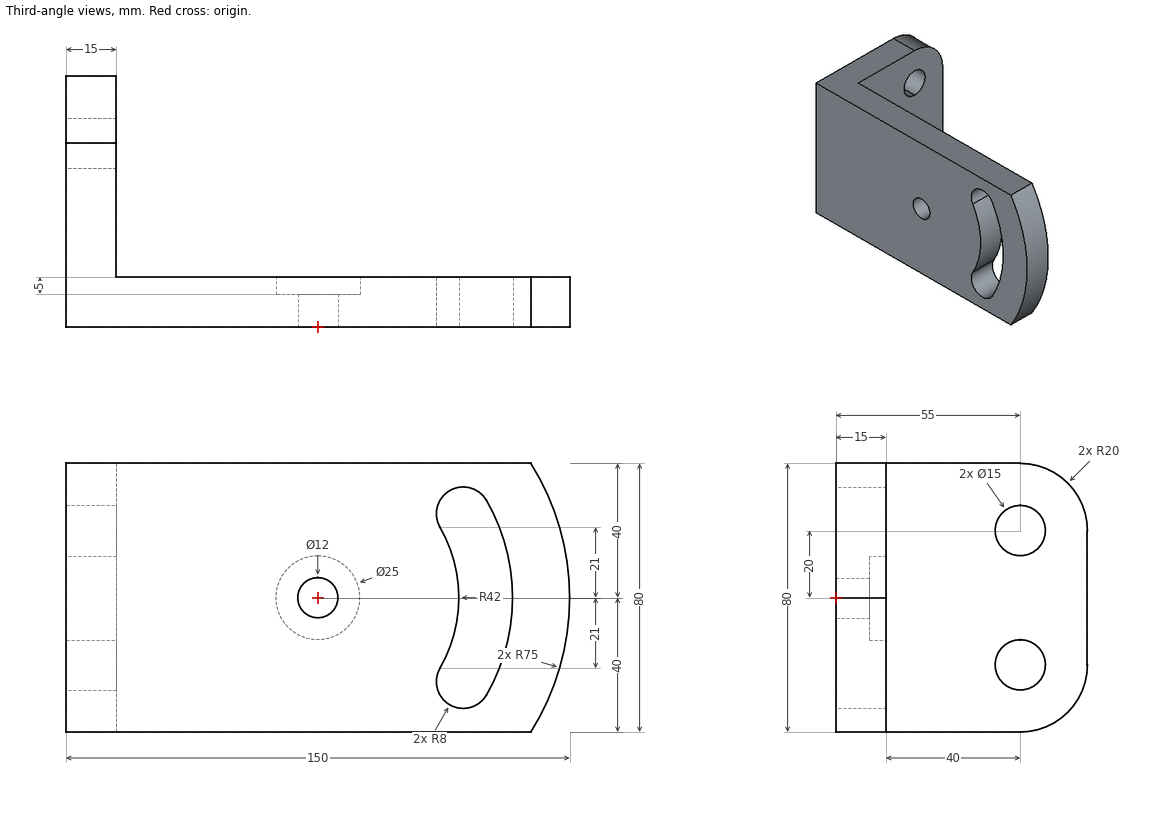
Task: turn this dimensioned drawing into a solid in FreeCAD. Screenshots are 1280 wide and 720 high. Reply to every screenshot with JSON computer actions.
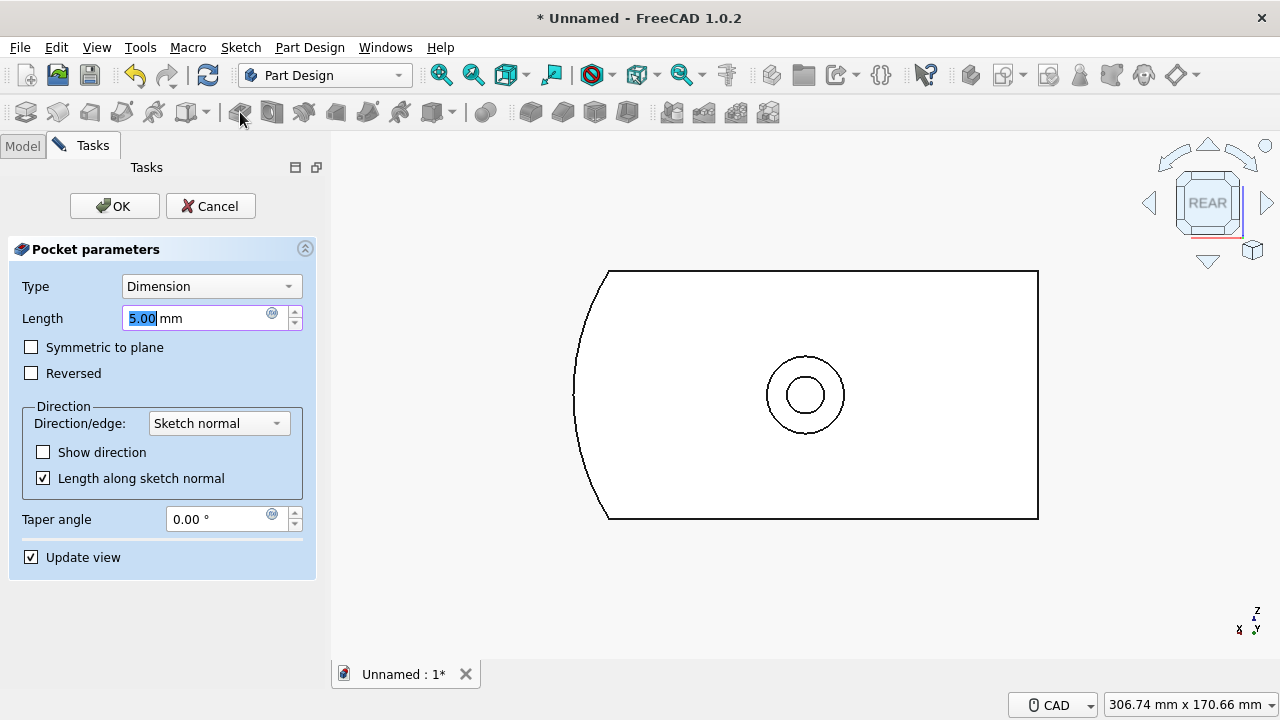
{"action": "type", "text": "5"}
{"action": "key", "text": "Tab"}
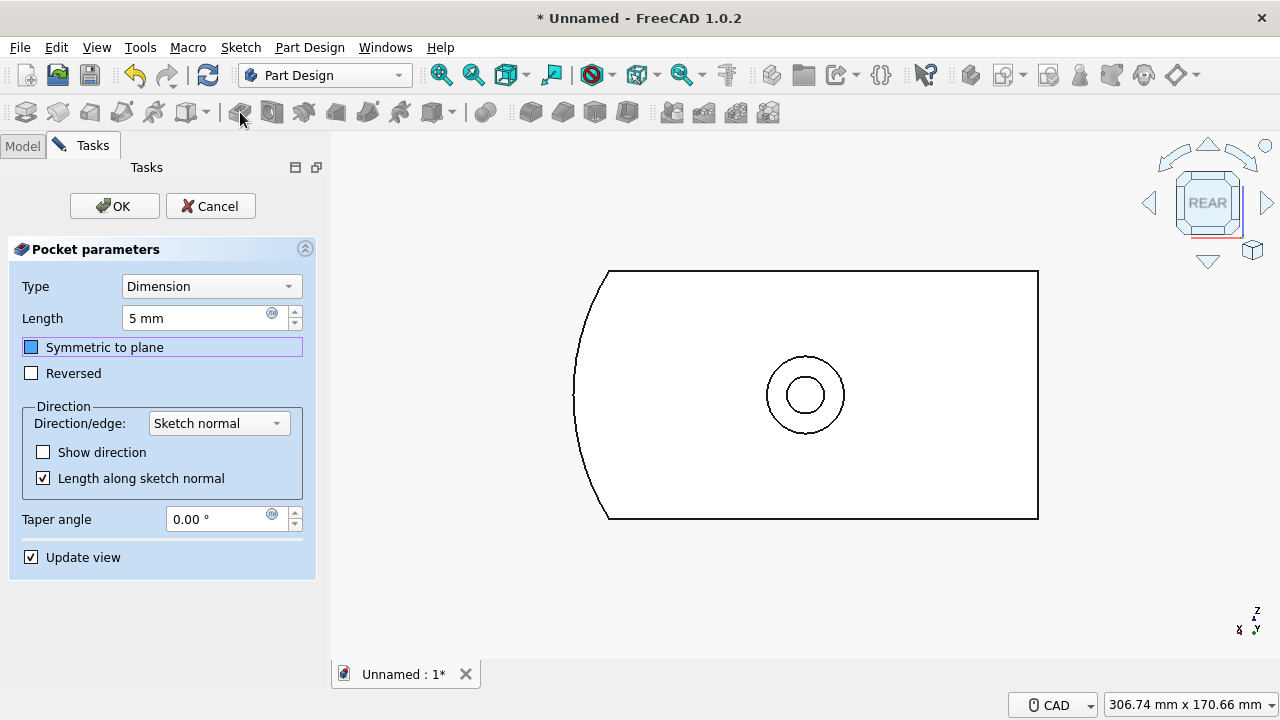
{"action": "left_click", "coordinate": [115, 206]}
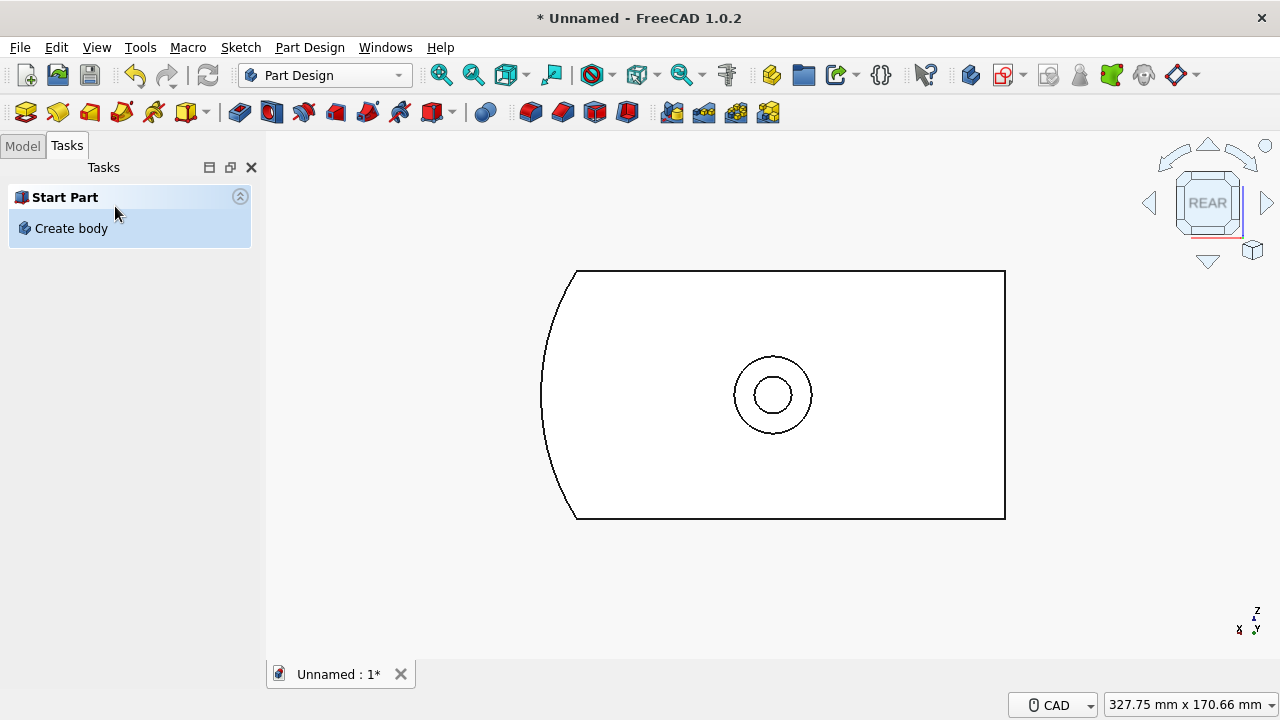
{"action": "left_click", "coordinate": [640, 394]}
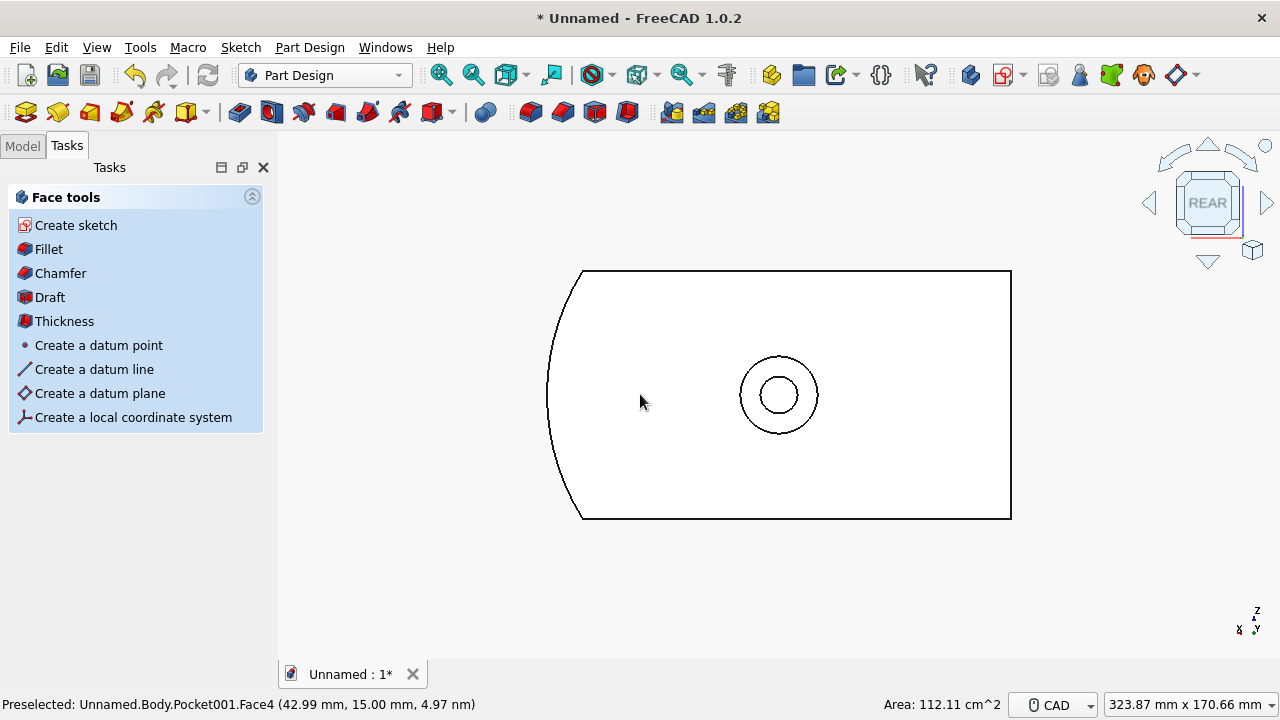
{"action": "left_click", "coordinate": [1004, 76]}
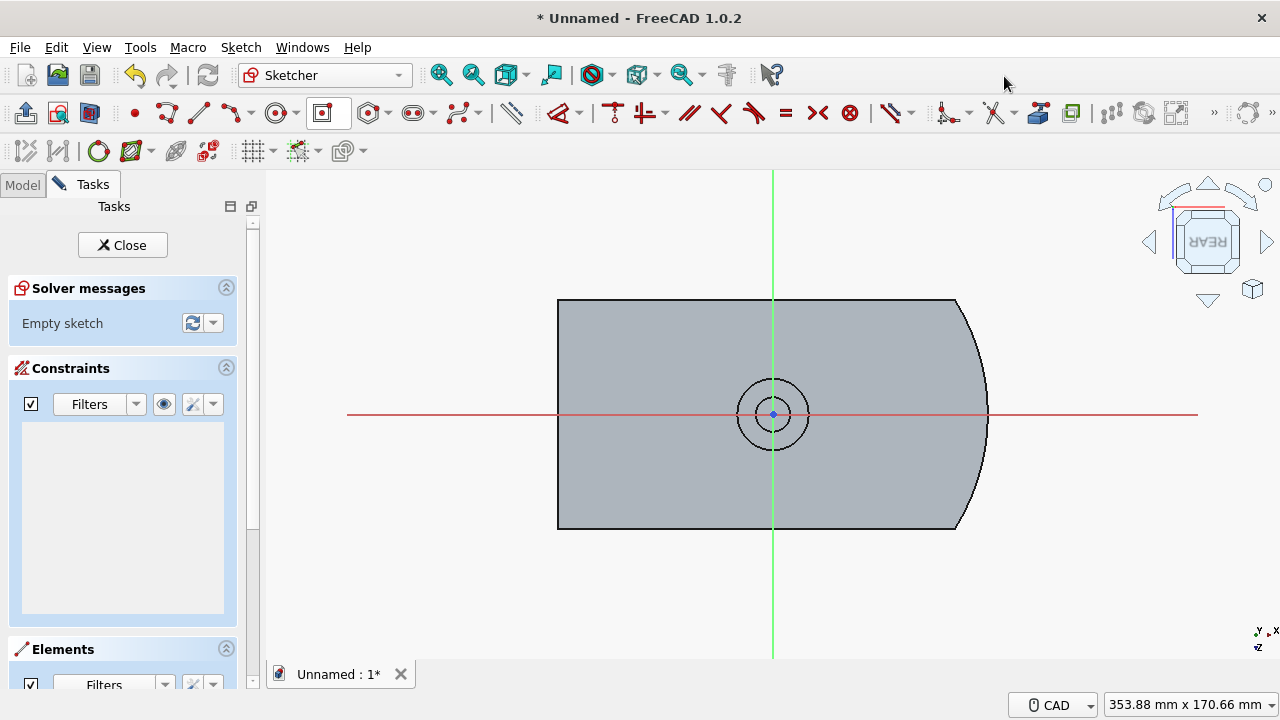
{"action": "scroll", "coordinate": [782, 414], "scroll_direction": "up", "scroll_amount": 11}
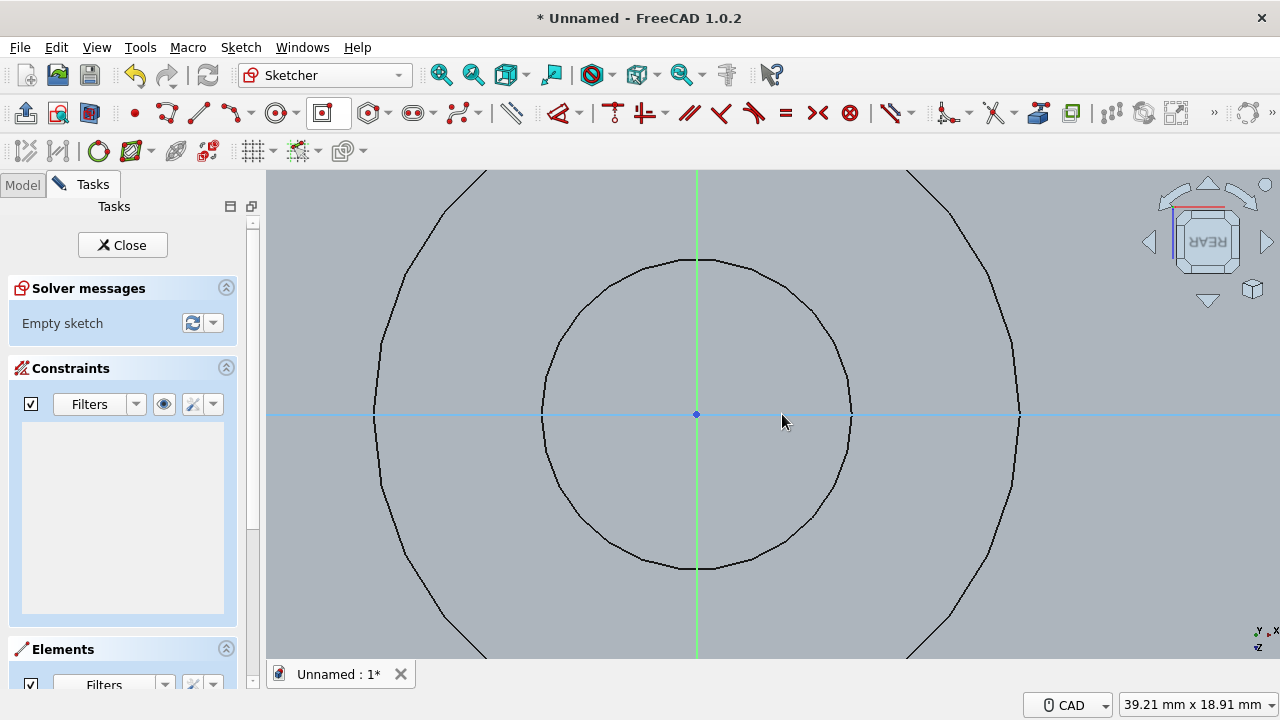
{"action": "left_click", "coordinate": [276, 114]}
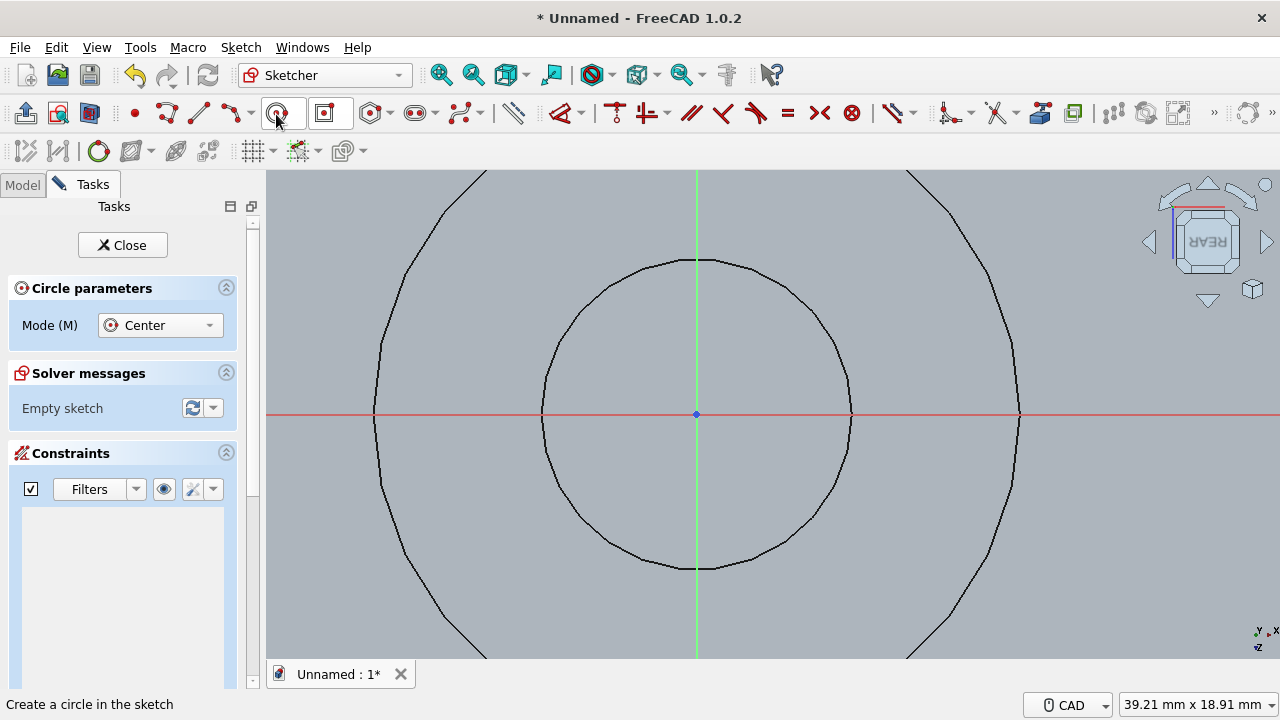
{"action": "left_click", "coordinate": [697, 414]}
{"action": "left_click", "coordinate": [806, 305]}
{"action": "key", "text": "Escape"}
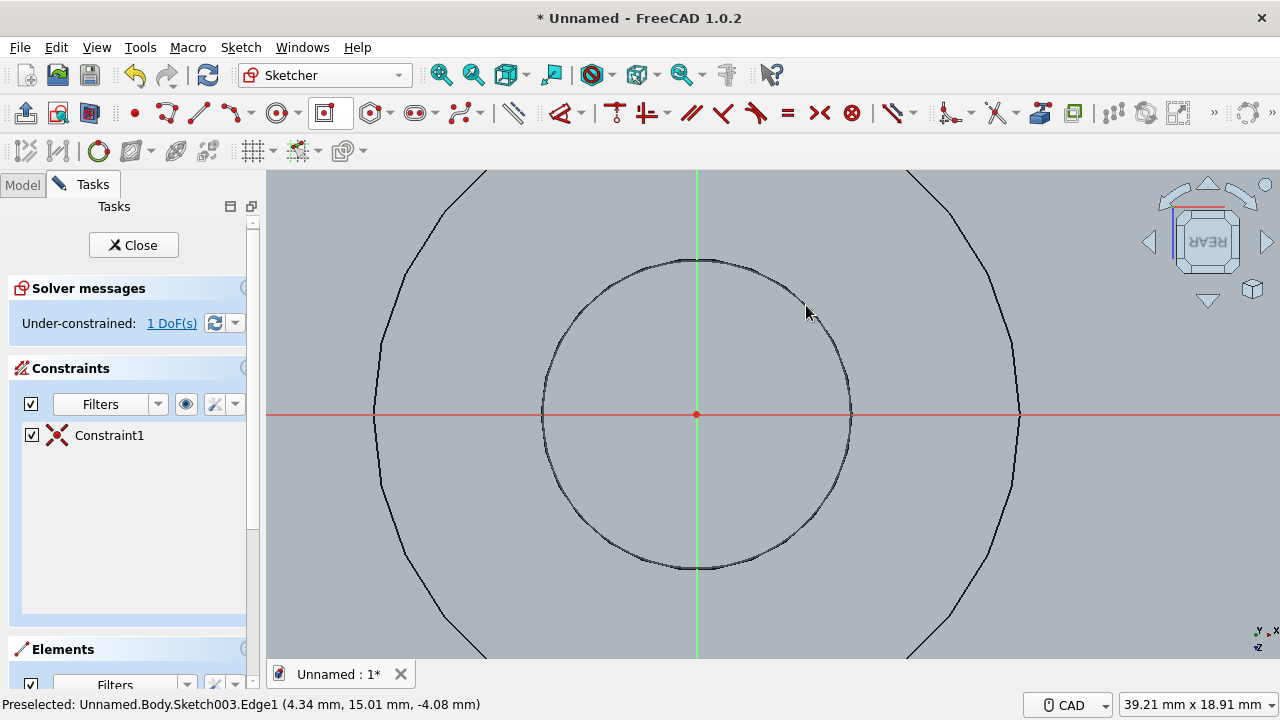
{"action": "left_click", "coordinate": [560, 114]}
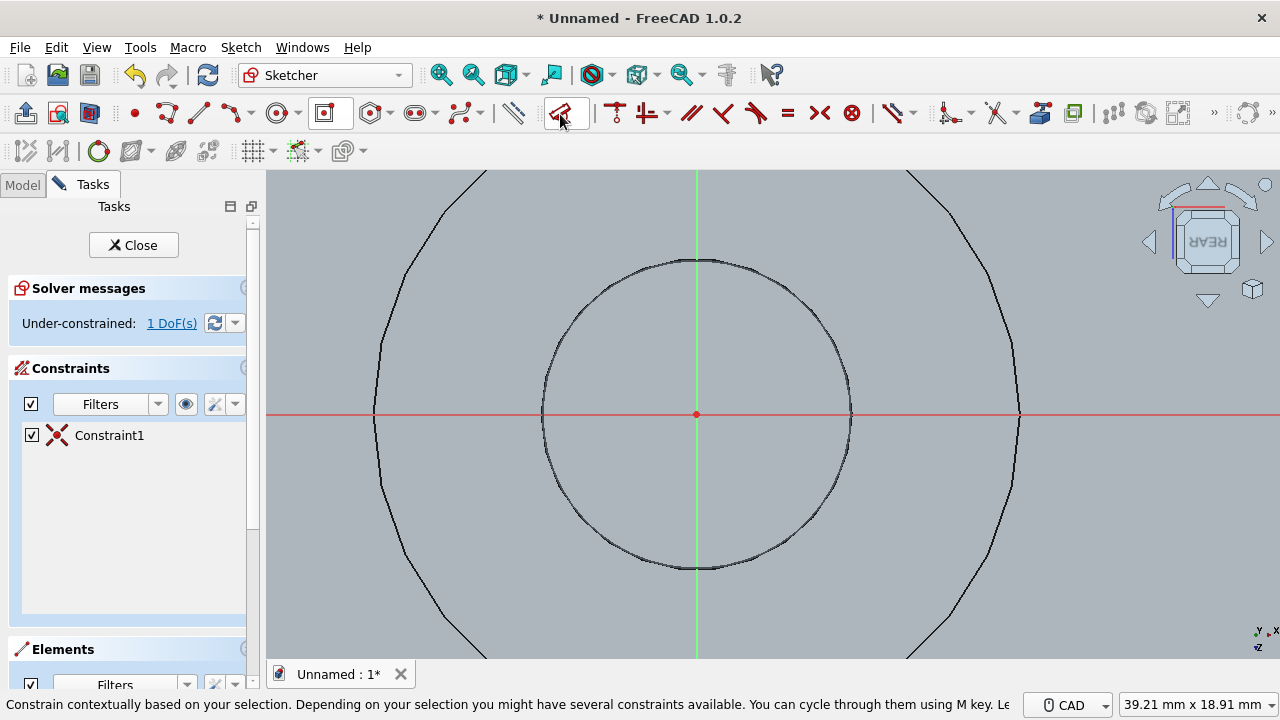
{"action": "left_click", "coordinate": [805, 305]}
{"action": "left_click", "coordinate": [828, 282]}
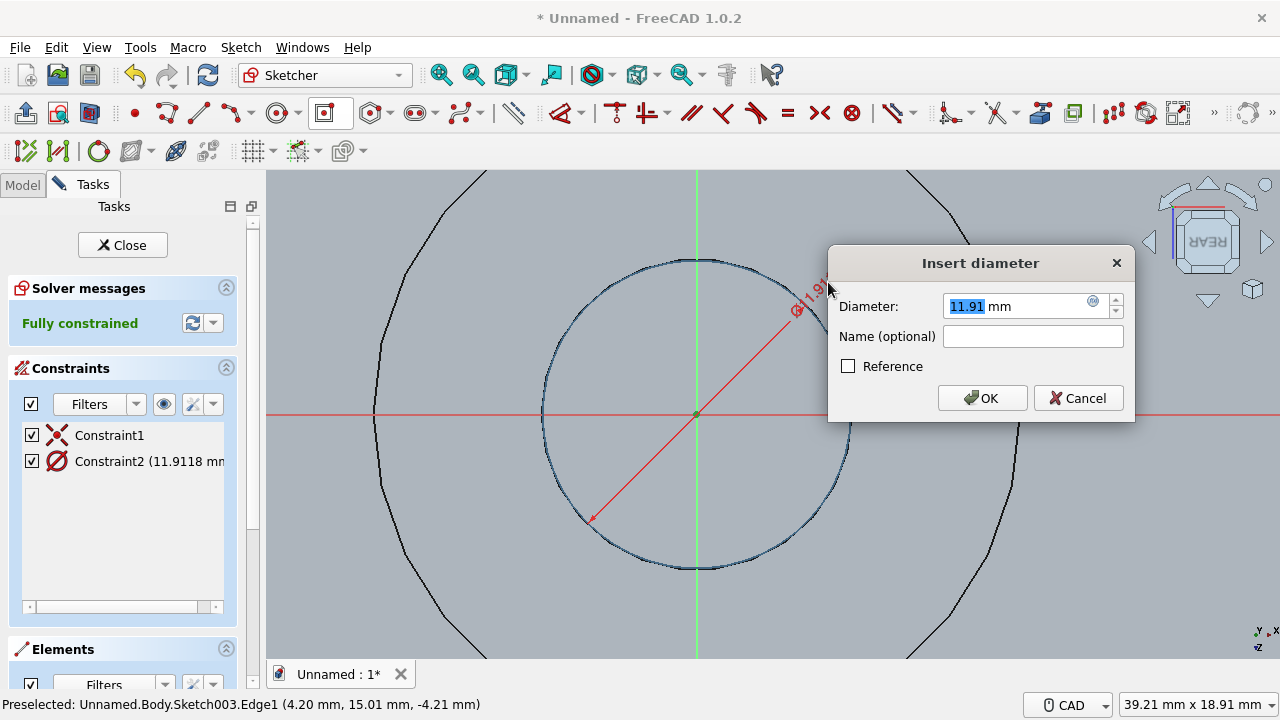
{"action": "type", "text": "12"}
{"action": "key", "text": "Return"}
{"action": "key", "text": "Escape"}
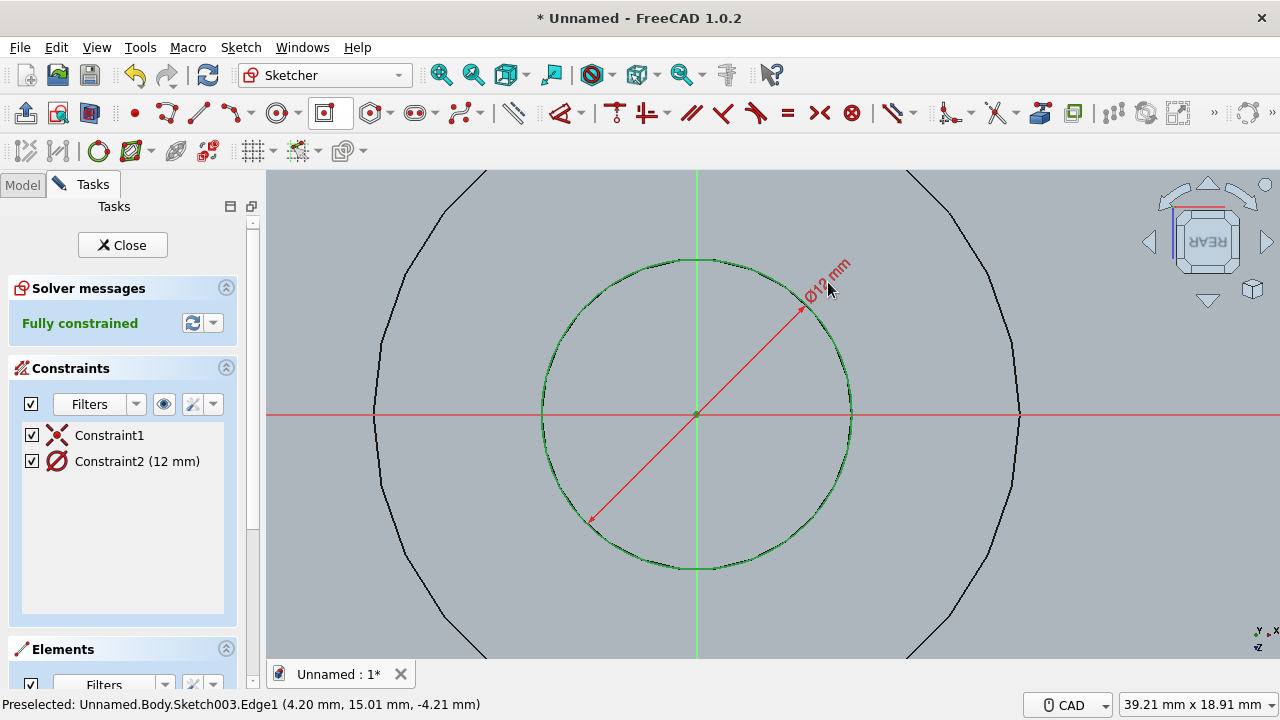
{"action": "left_click", "coordinate": [123, 245]}